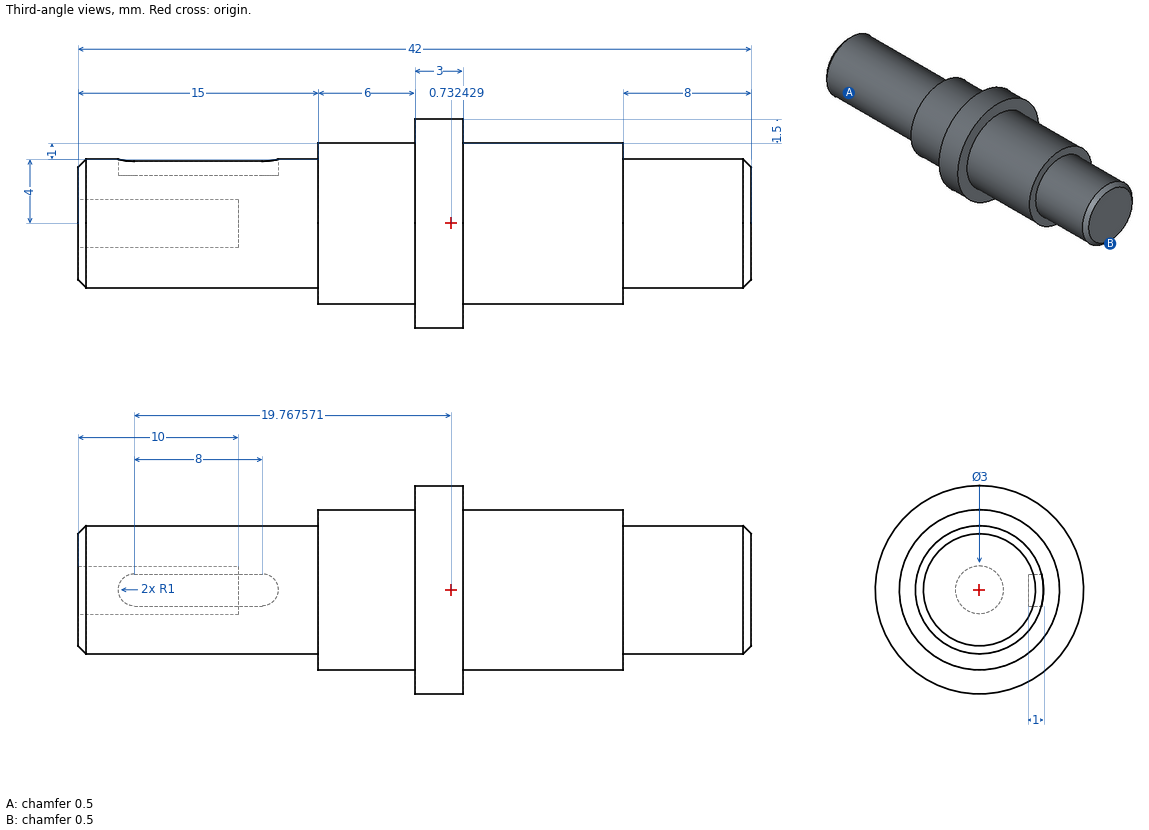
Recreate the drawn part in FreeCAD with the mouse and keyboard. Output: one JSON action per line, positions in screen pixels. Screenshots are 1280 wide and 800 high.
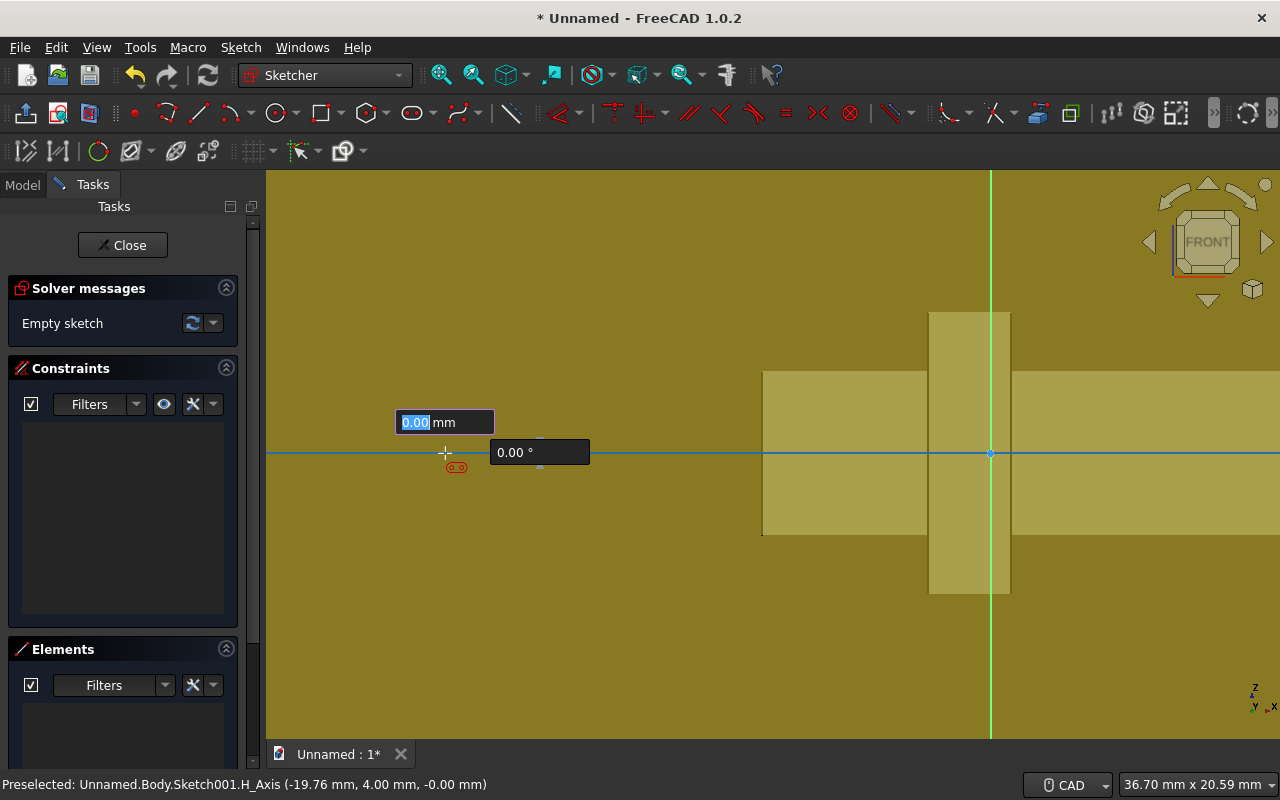
{"action": "left_click", "coordinate": [666, 444]}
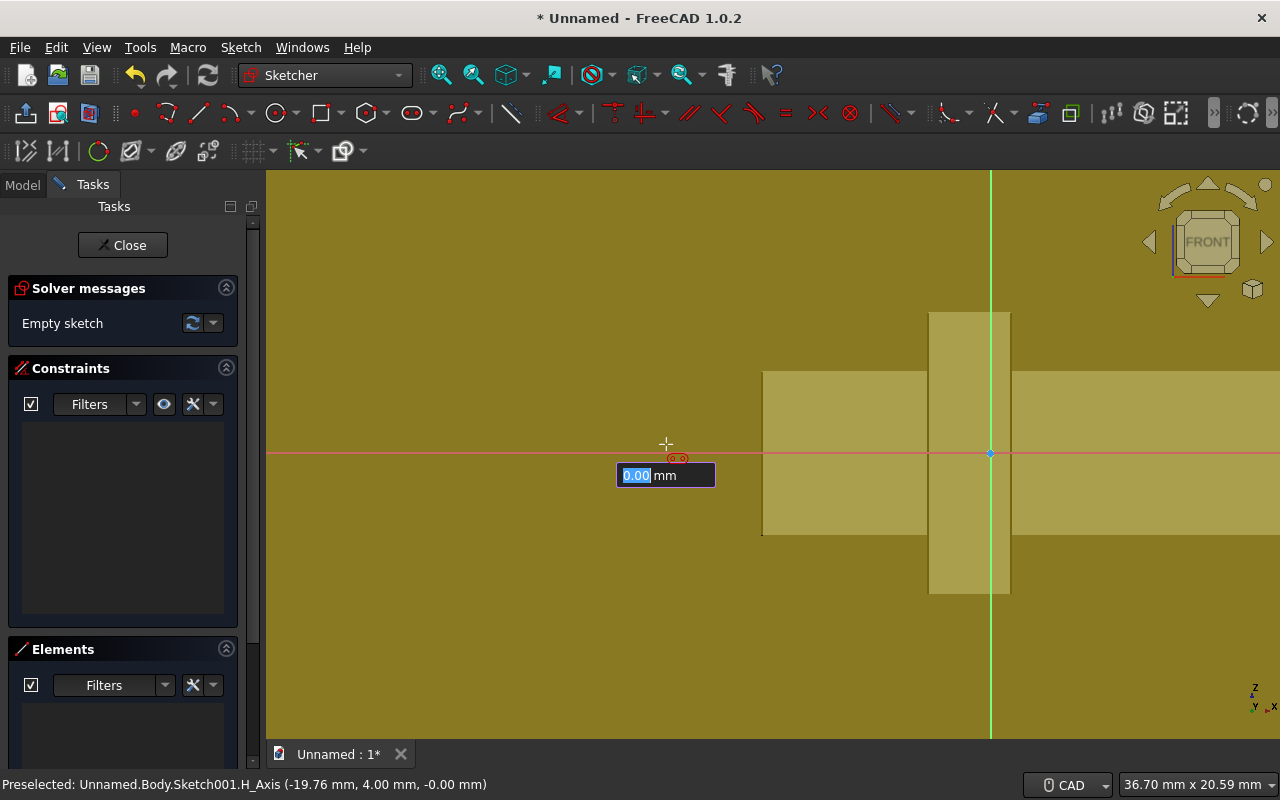
{"action": "left_click", "coordinate": [555, 481]}
{"action": "key", "text": "Escape"}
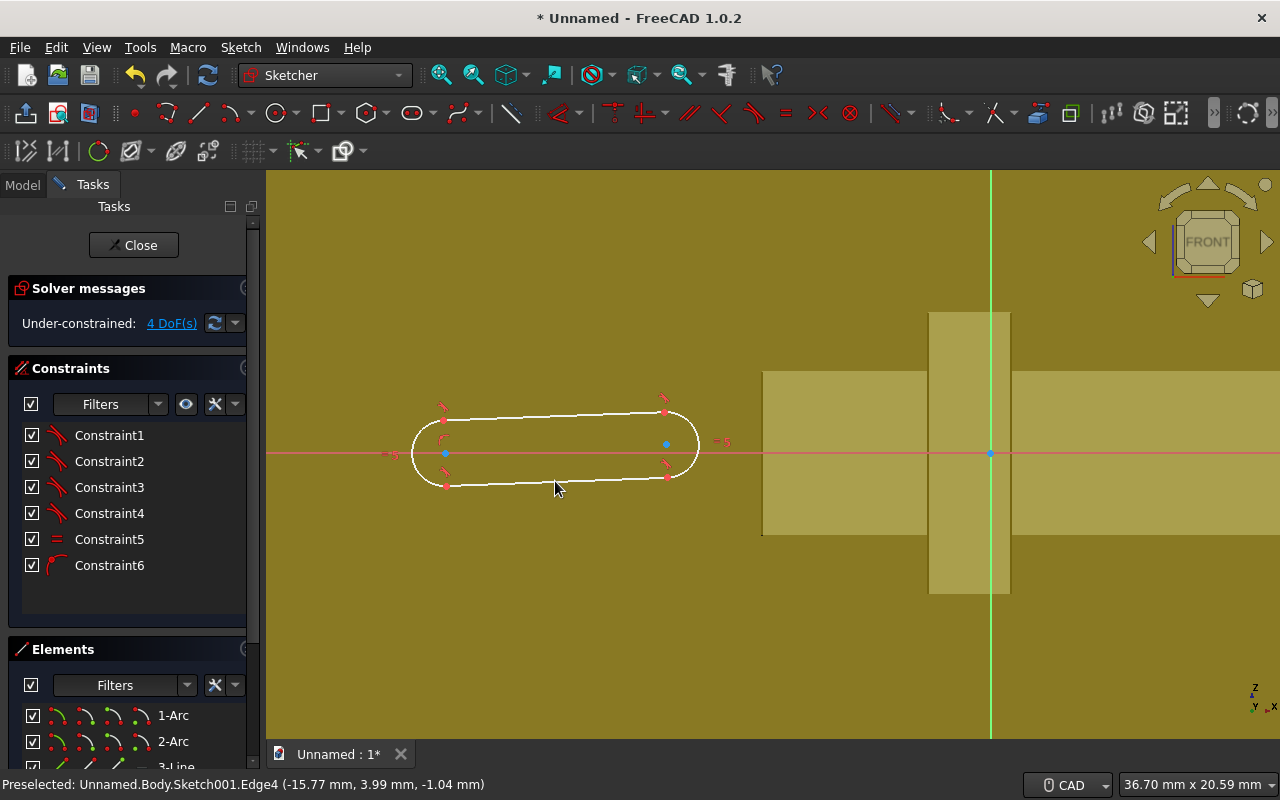
{"action": "left_click", "coordinate": [510, 418]}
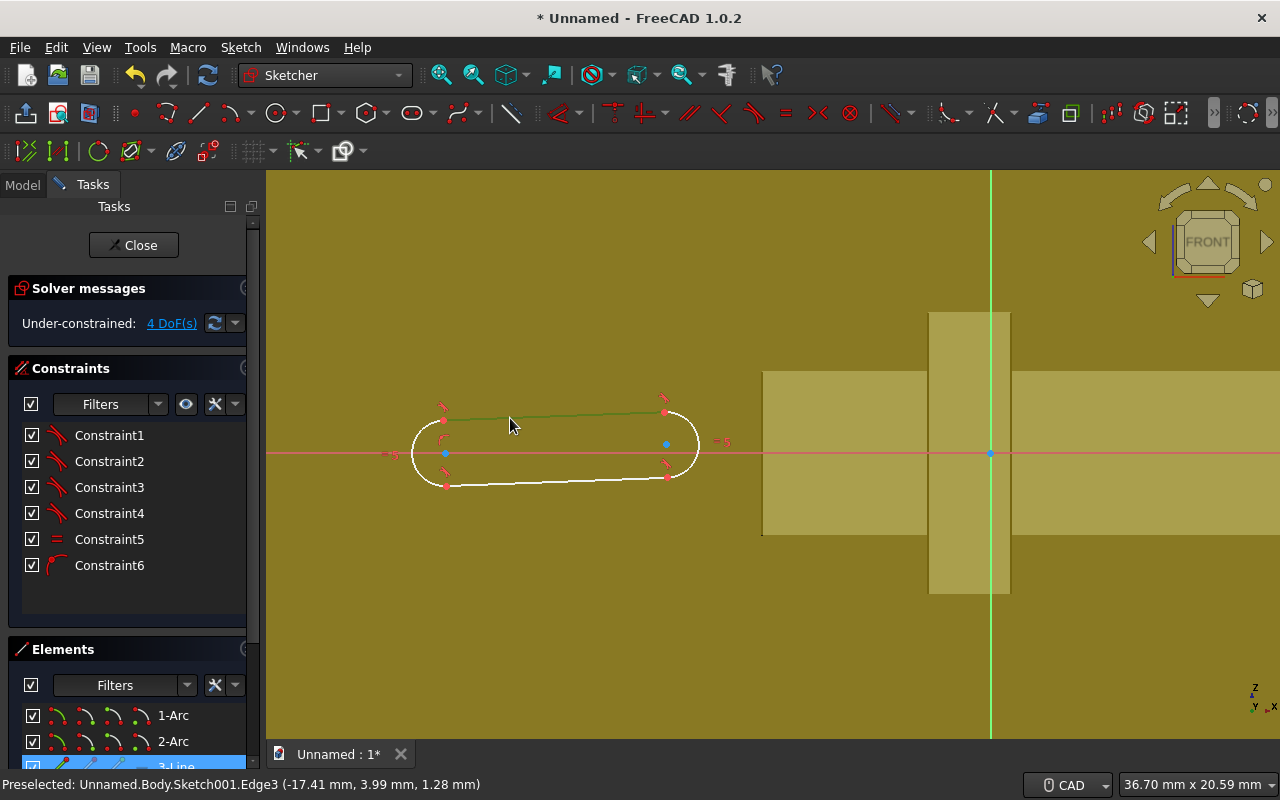
{"action": "left_click", "coordinate": [668, 114]}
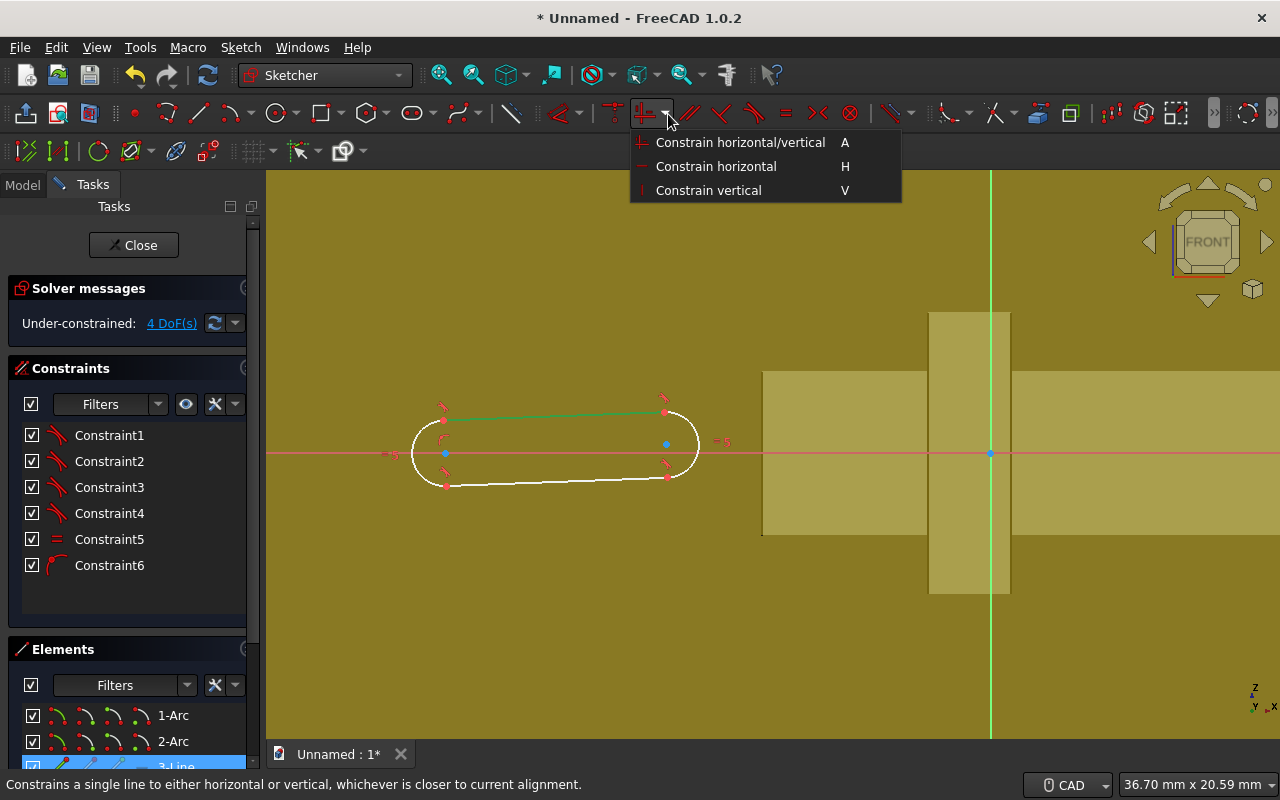
{"action": "left_click", "coordinate": [766, 166]}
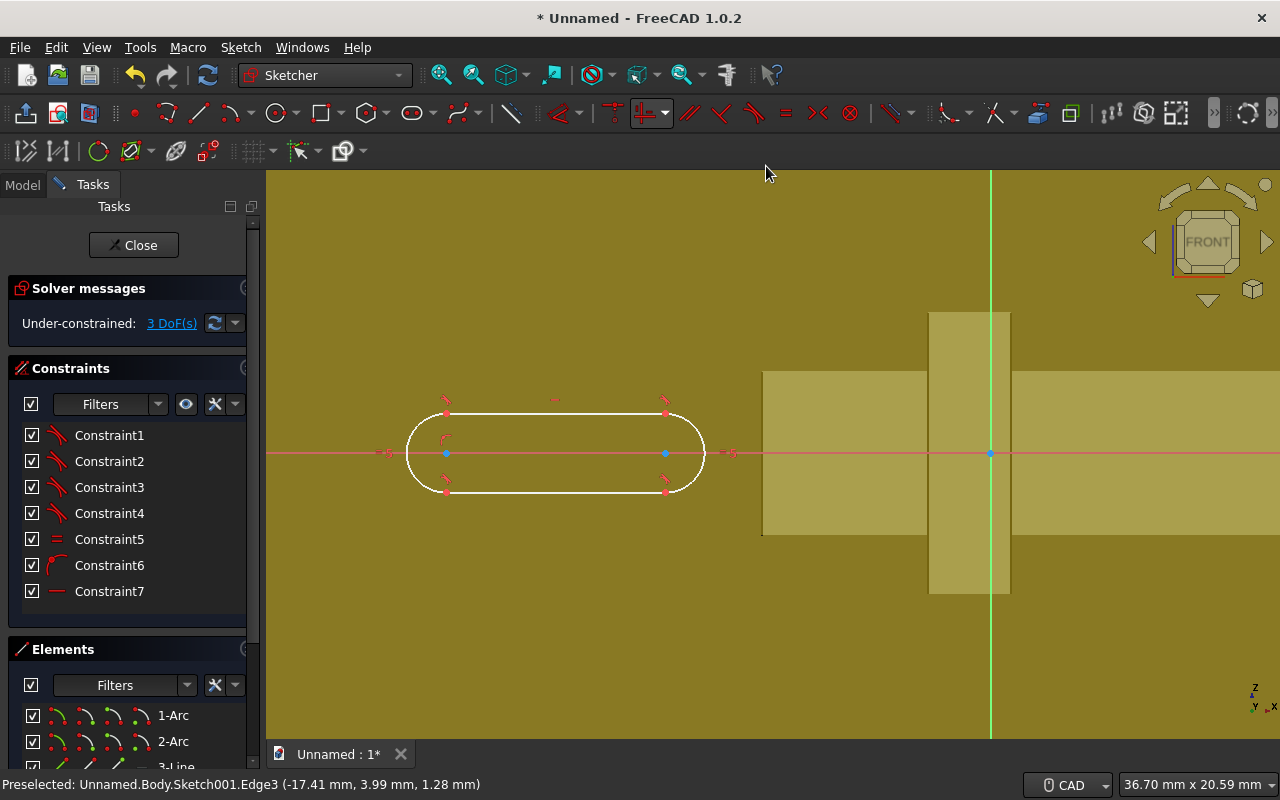
{"action": "left_click", "coordinate": [558, 114]}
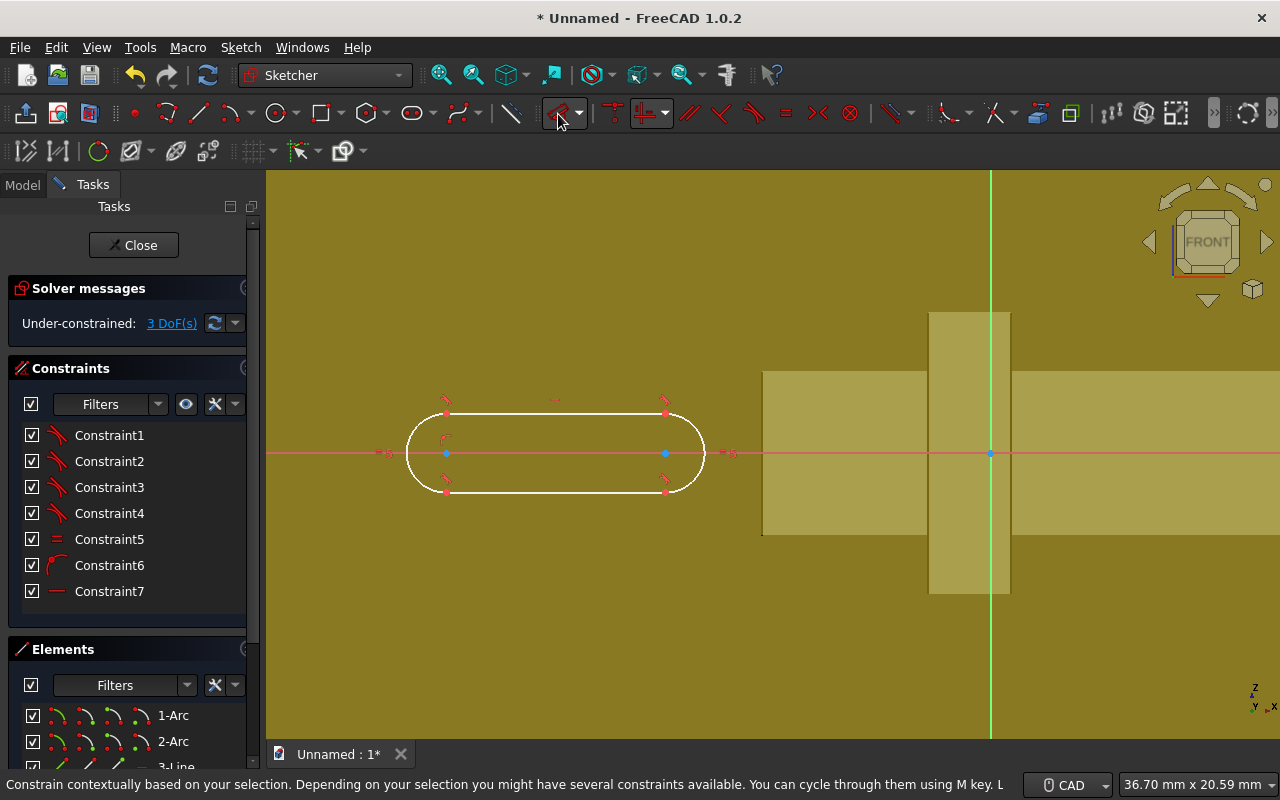
{"action": "scroll", "coordinate": [414, 430], "scroll_direction": "up", "scroll_amount": 2}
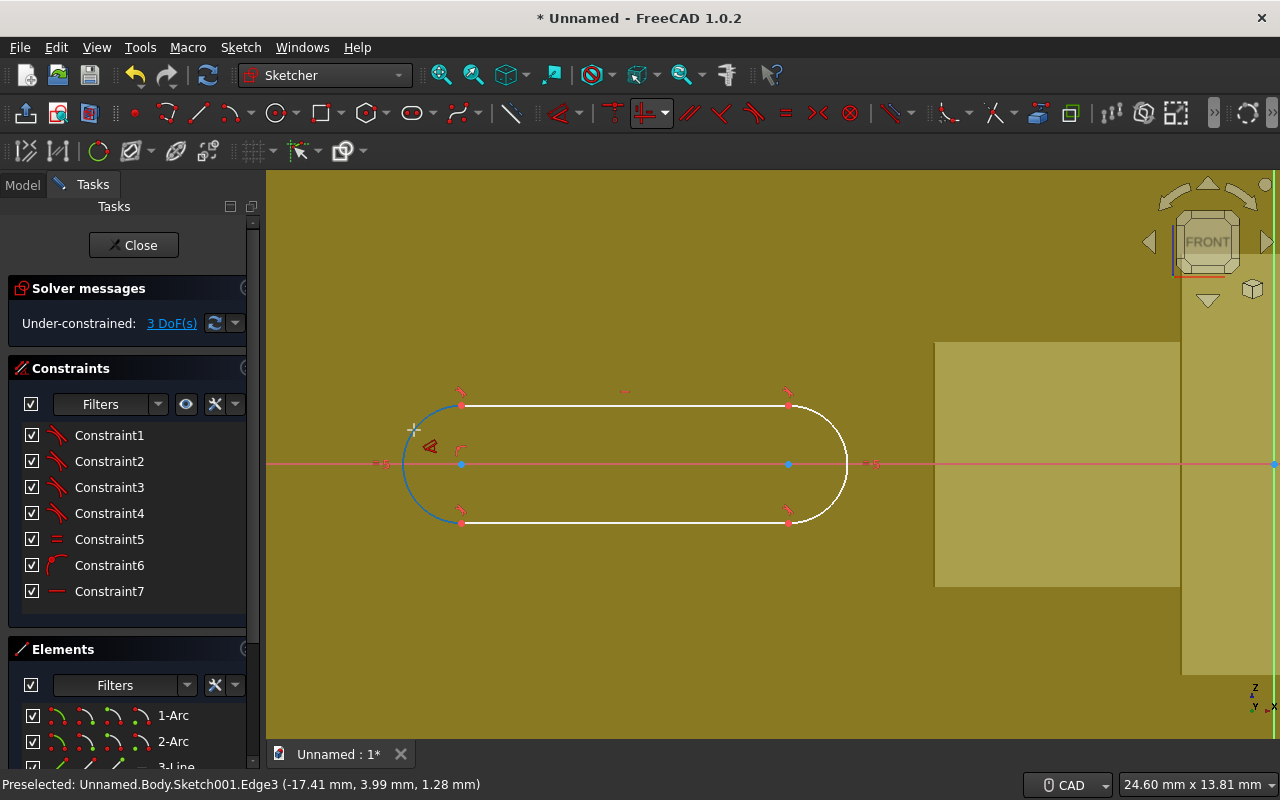
{"action": "left_click", "coordinate": [414, 430]}
{"action": "left_click", "coordinate": [388, 411]}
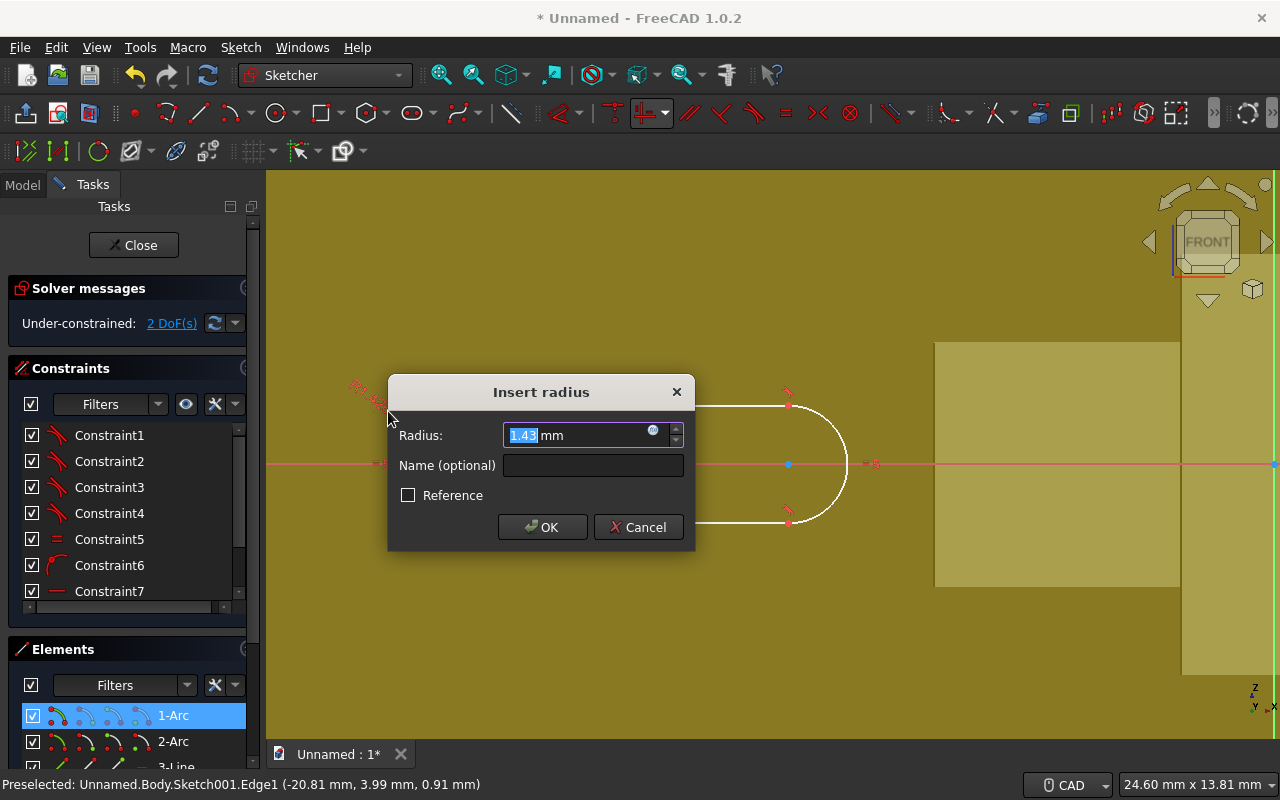
{"action": "type", "text": "1"}
{"action": "key", "text": "Return"}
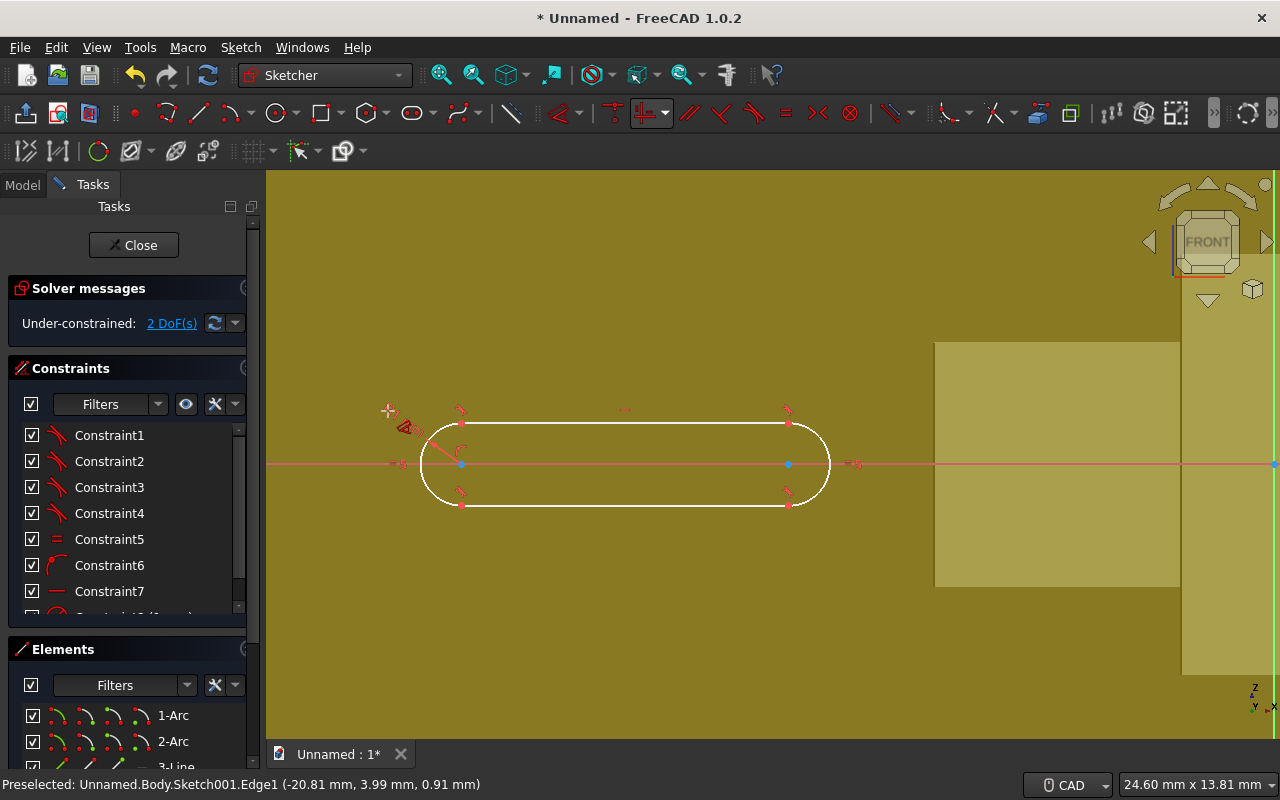
{"action": "left_click", "coordinate": [560, 423]}
{"action": "left_click", "coordinate": [625, 389]}